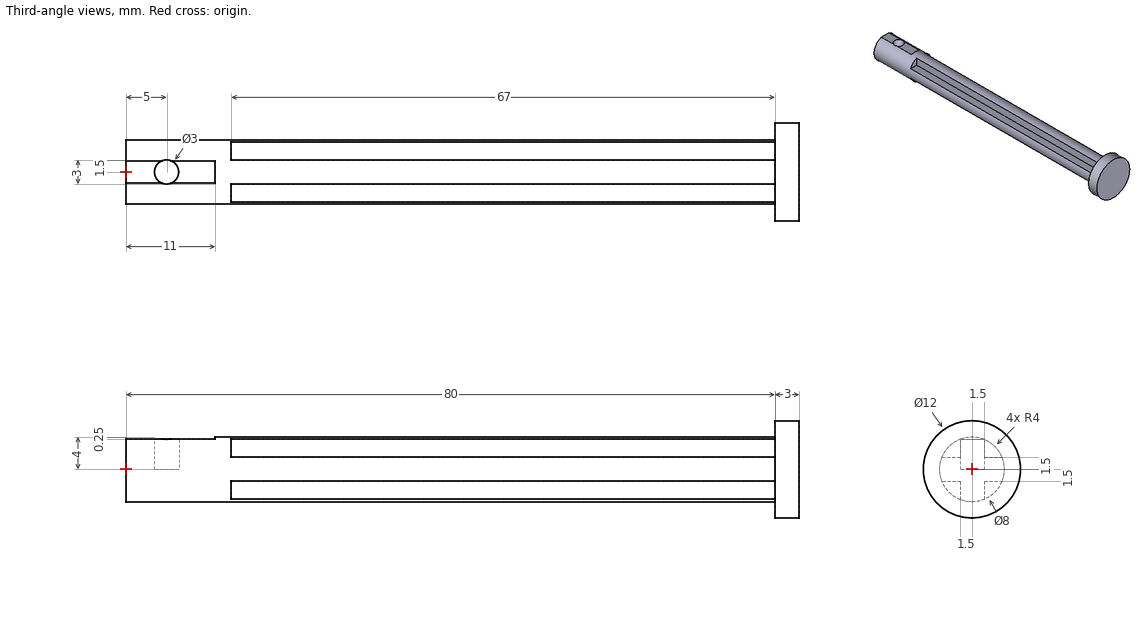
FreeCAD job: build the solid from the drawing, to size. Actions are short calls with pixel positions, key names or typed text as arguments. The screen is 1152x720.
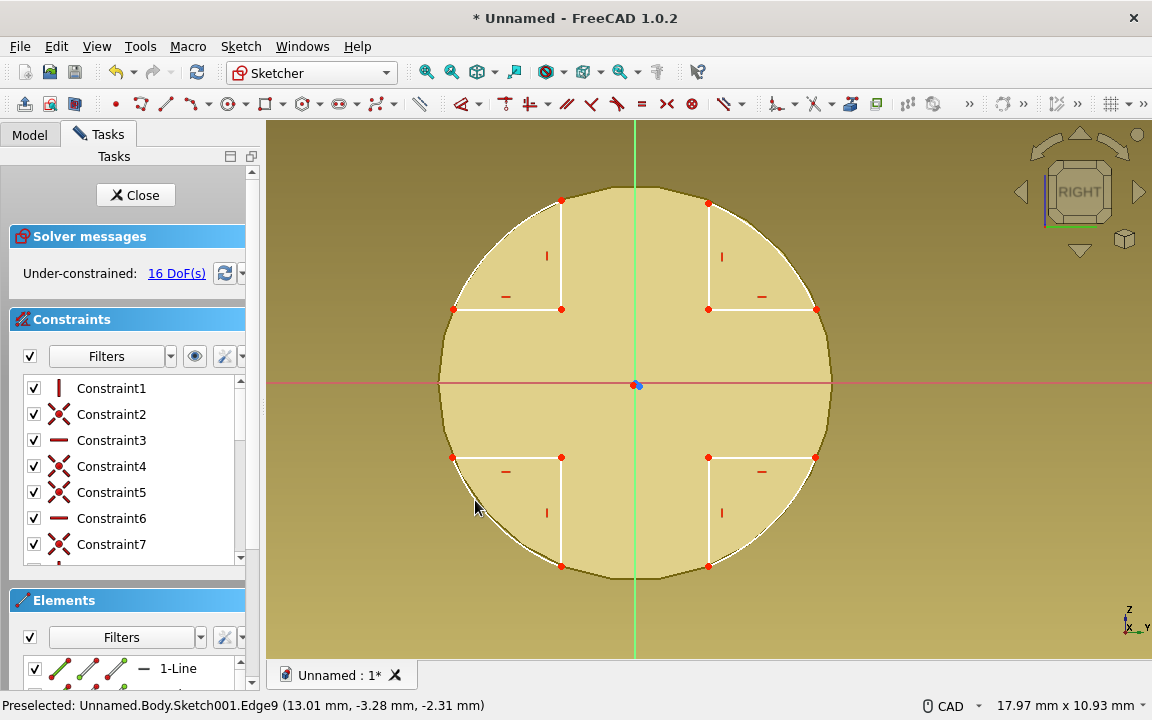
click(793, 269)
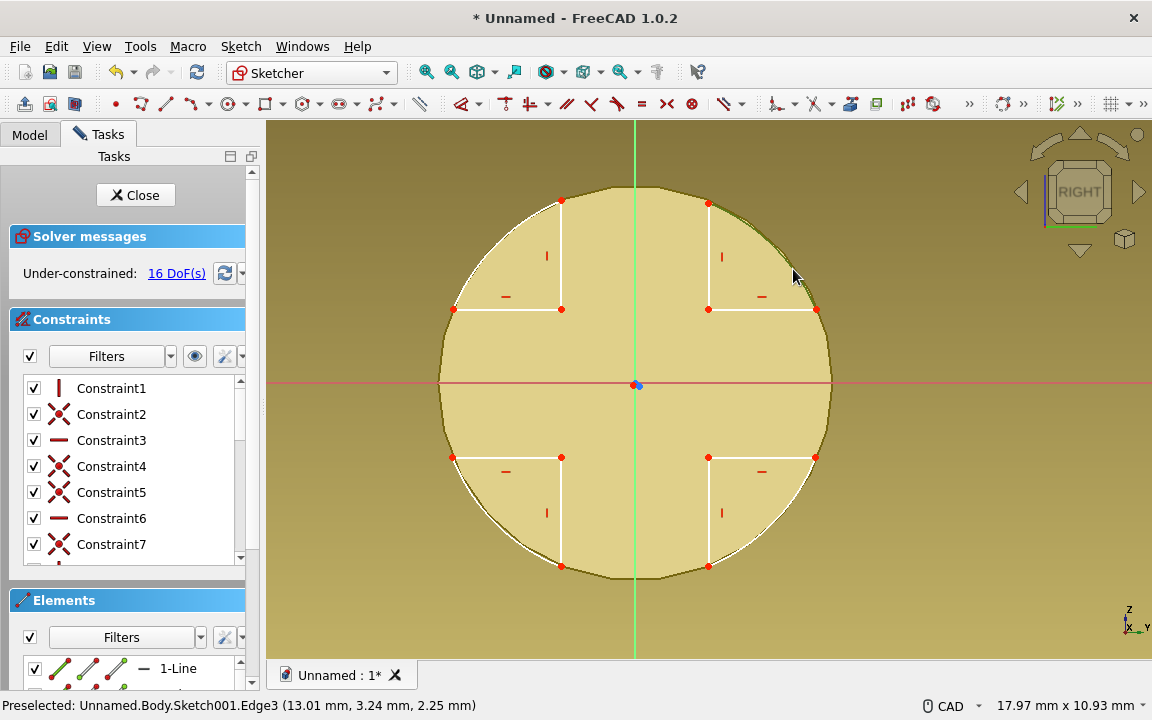
click(520, 224)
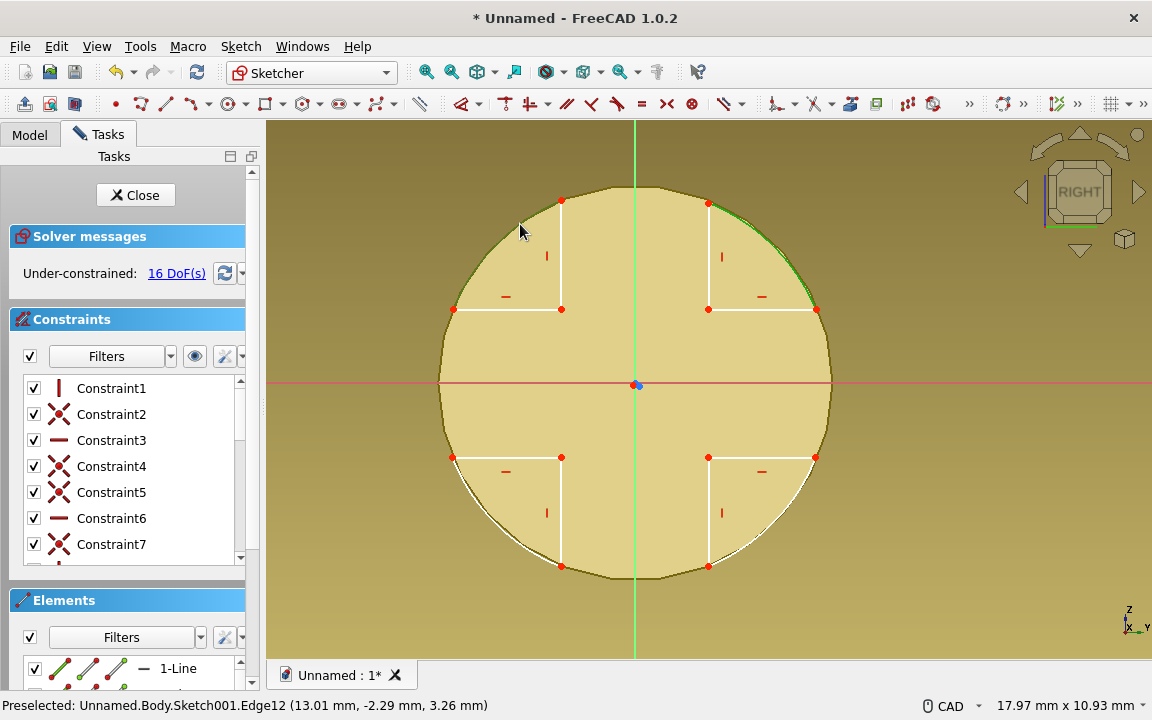
key(c)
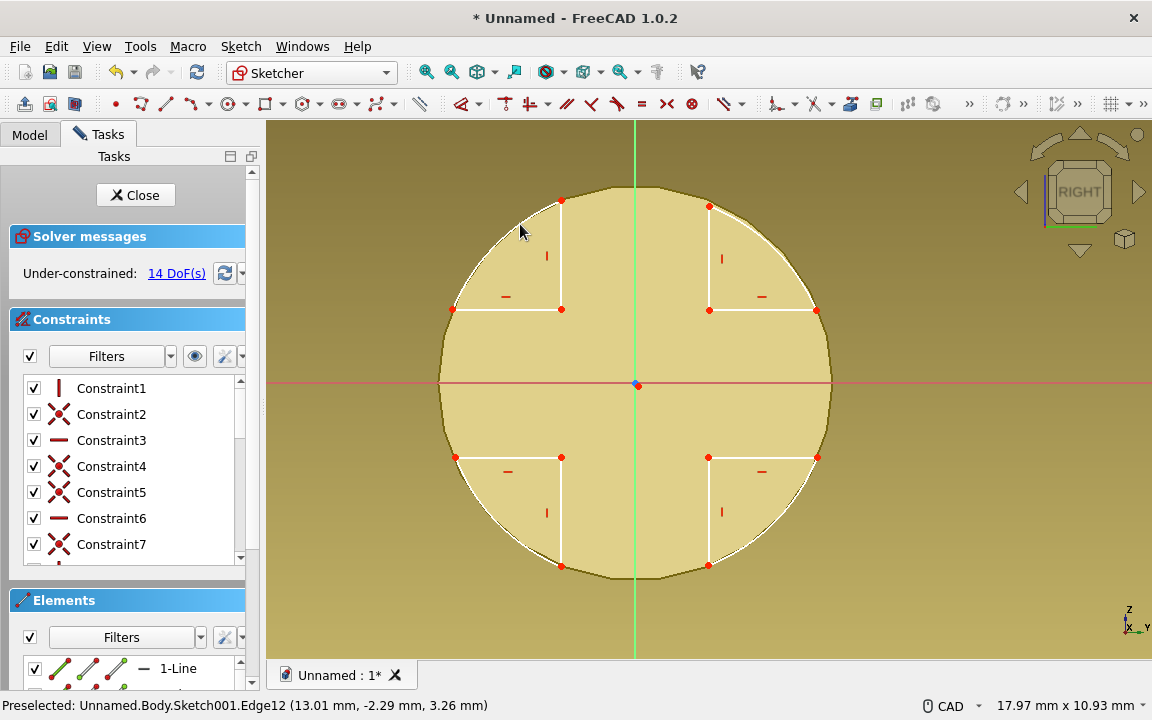
drag(625, 373, 648, 396)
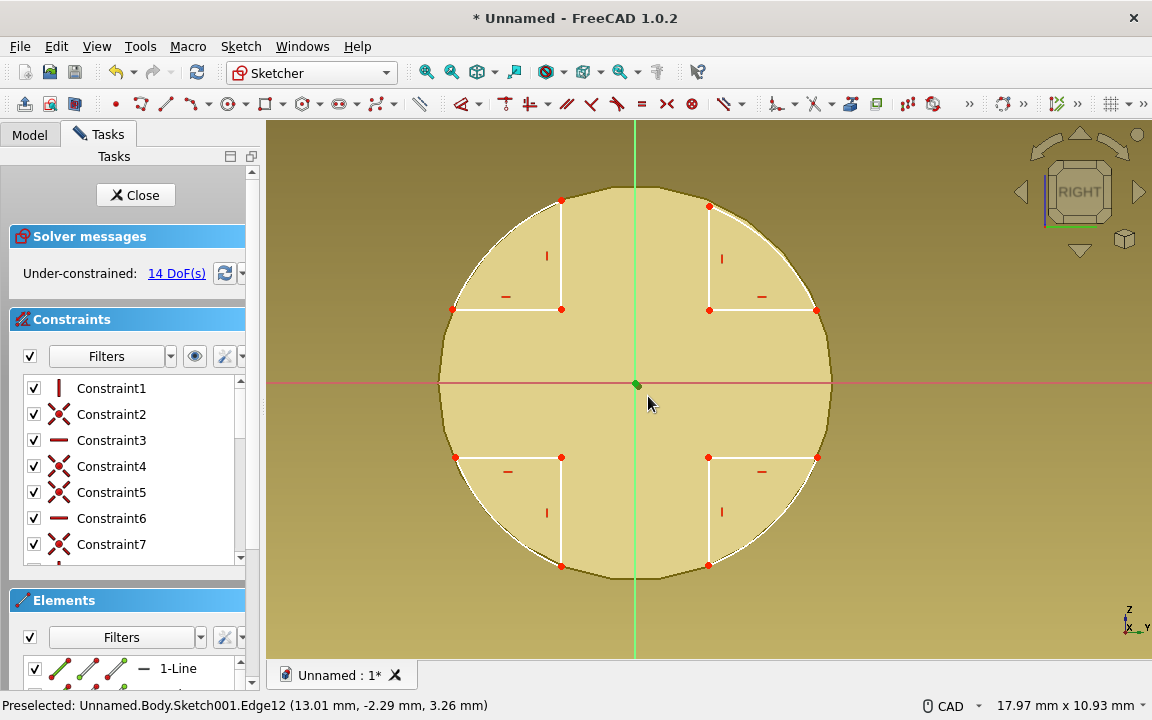
key(c)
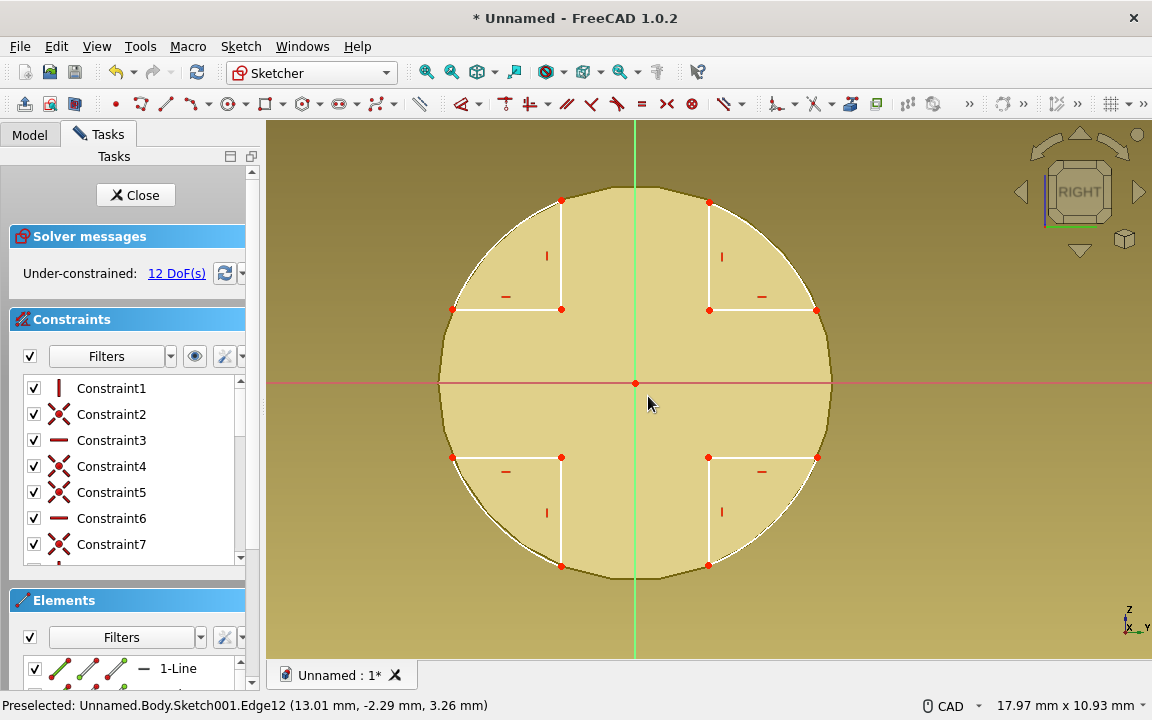
click(794, 269)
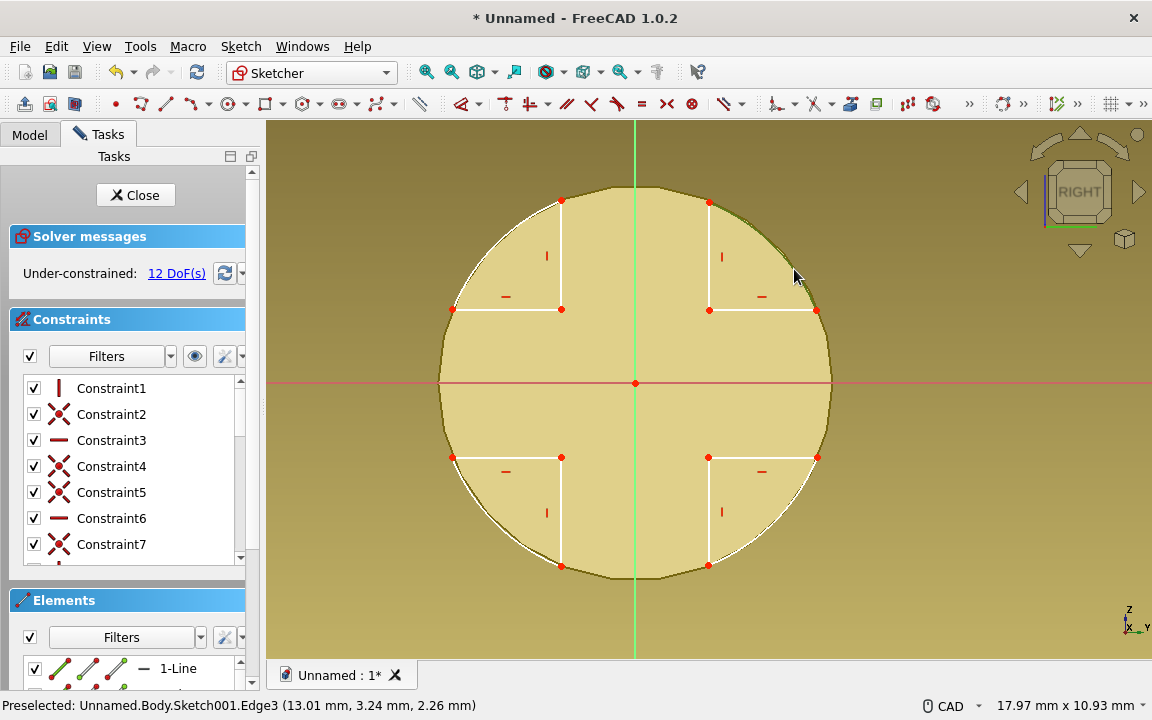
click(750, 543)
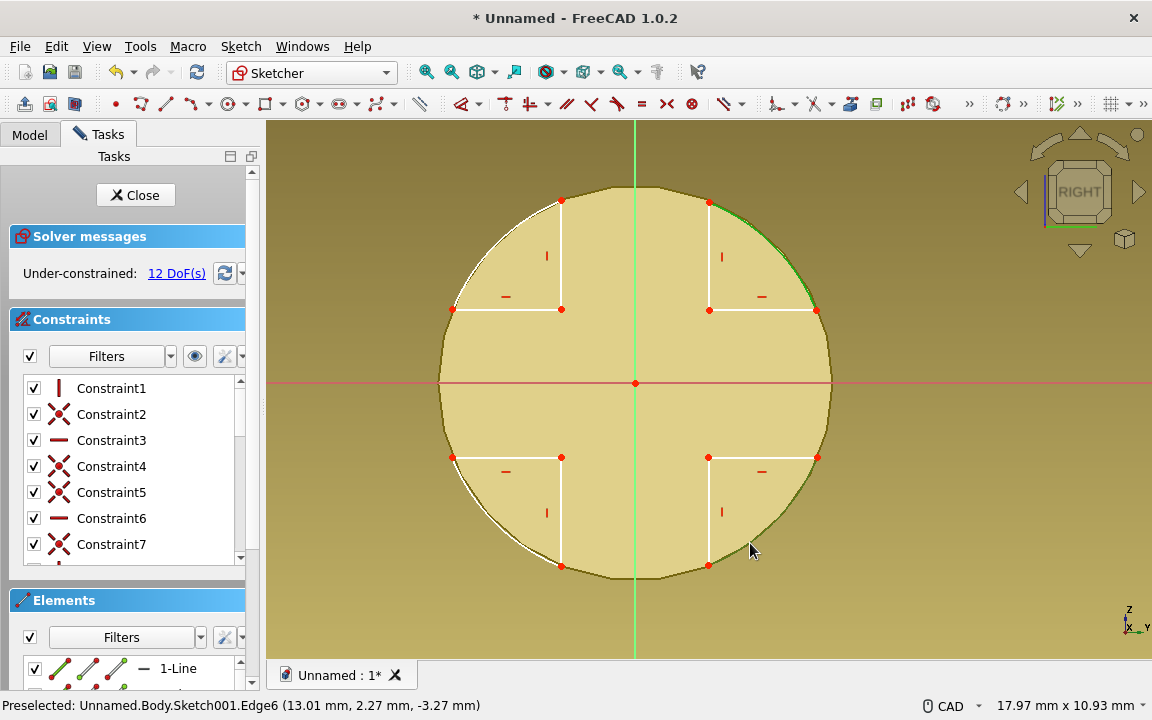
click(475, 499)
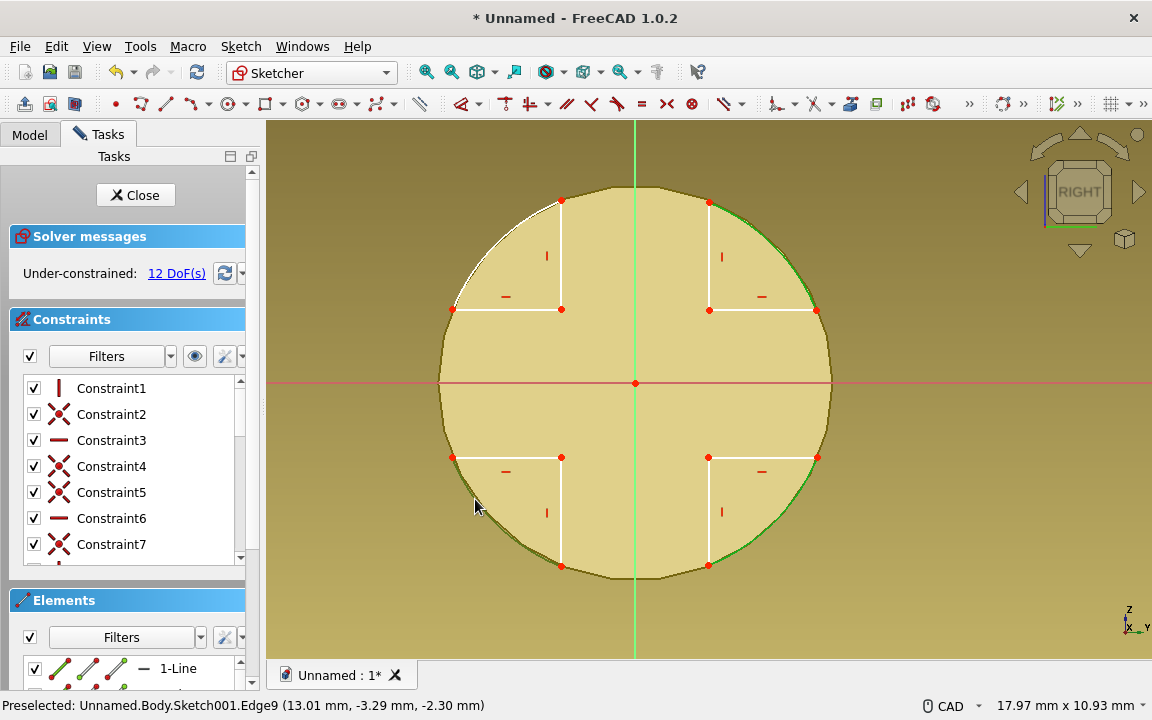
click(520, 224)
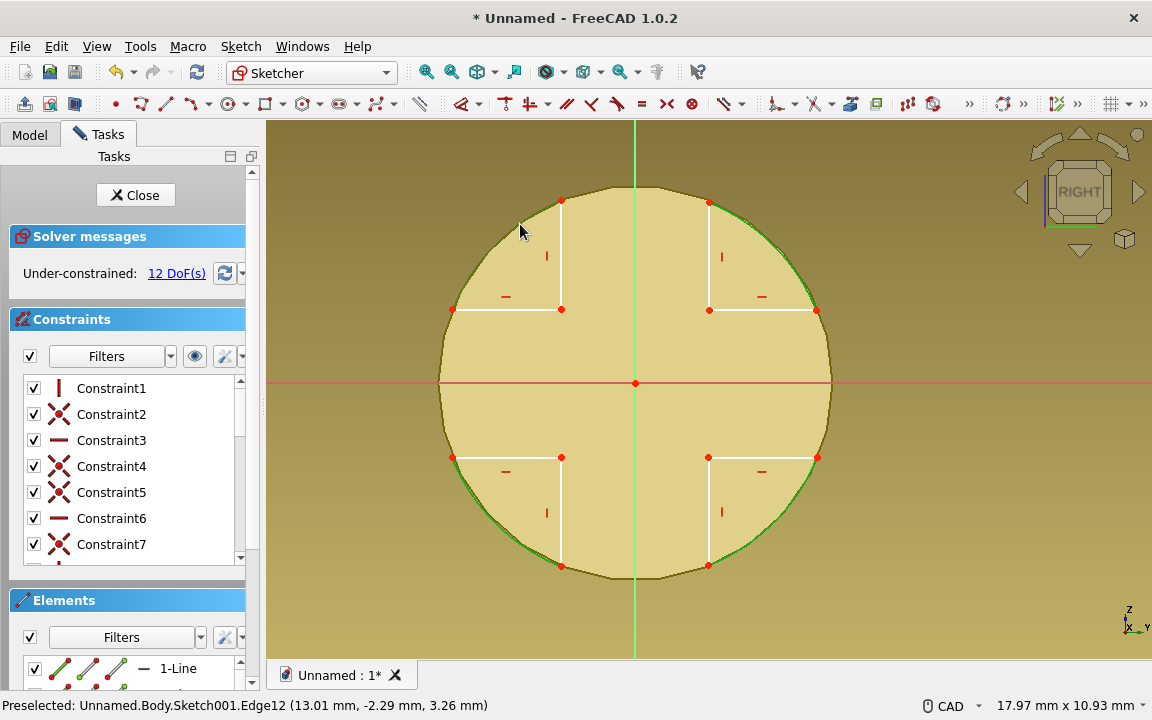
key(e)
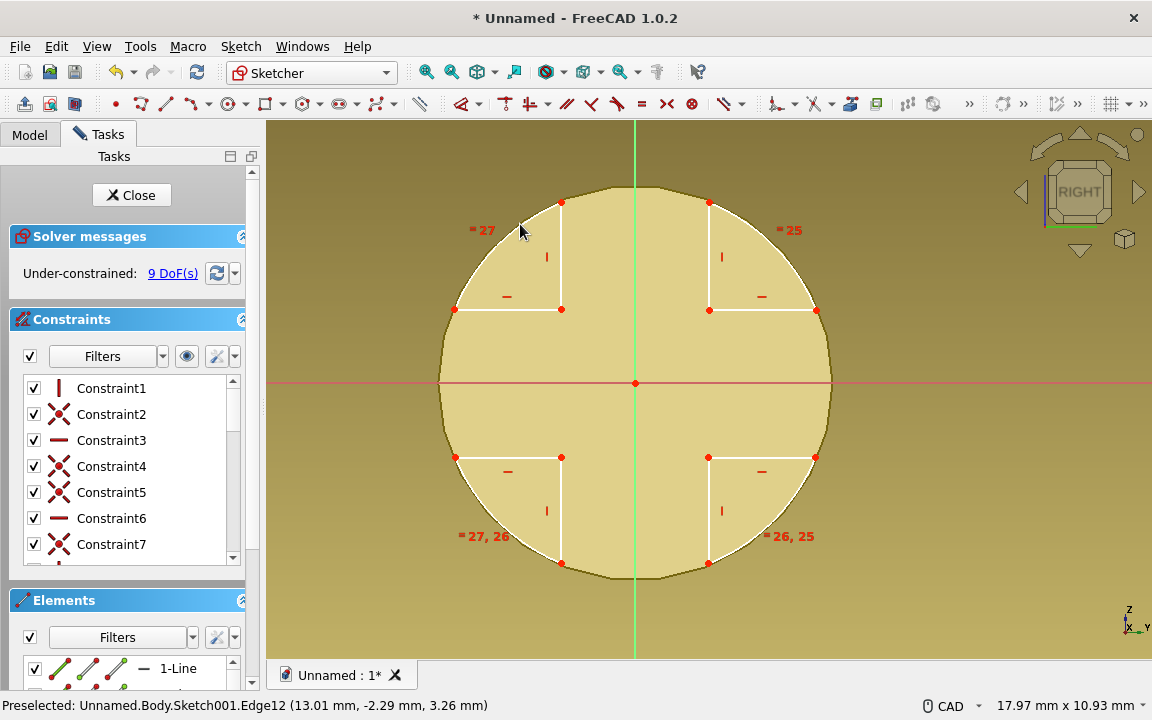
click(794, 269)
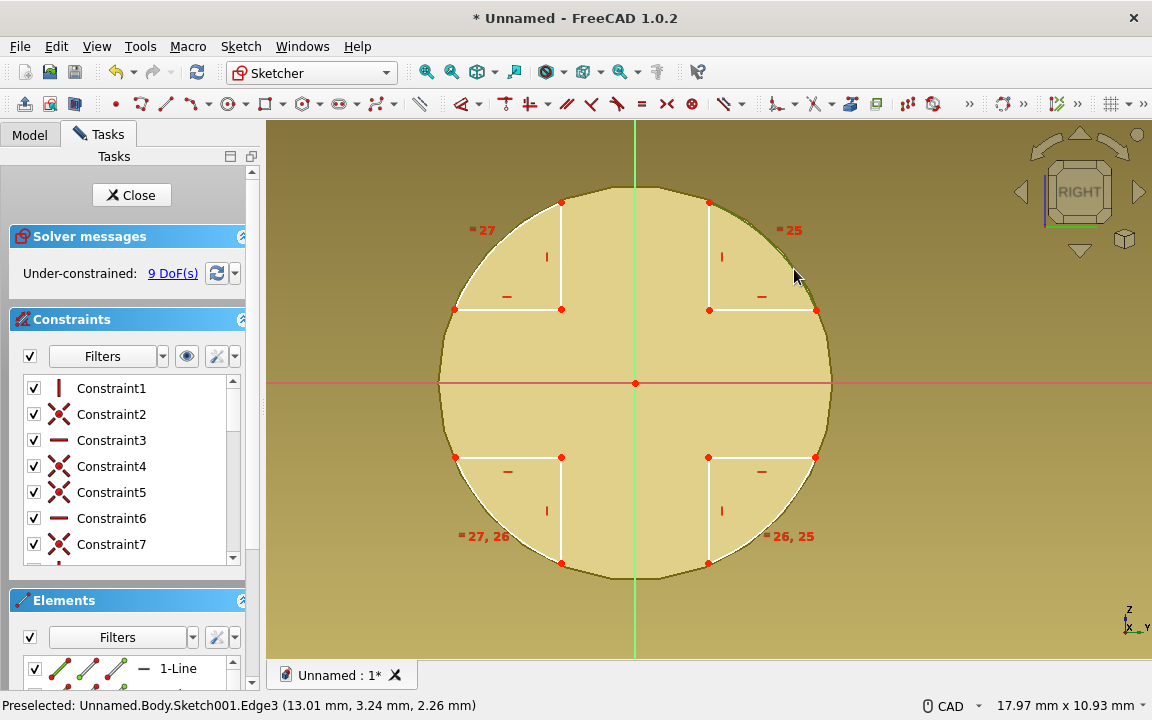
key(k)
key(r)